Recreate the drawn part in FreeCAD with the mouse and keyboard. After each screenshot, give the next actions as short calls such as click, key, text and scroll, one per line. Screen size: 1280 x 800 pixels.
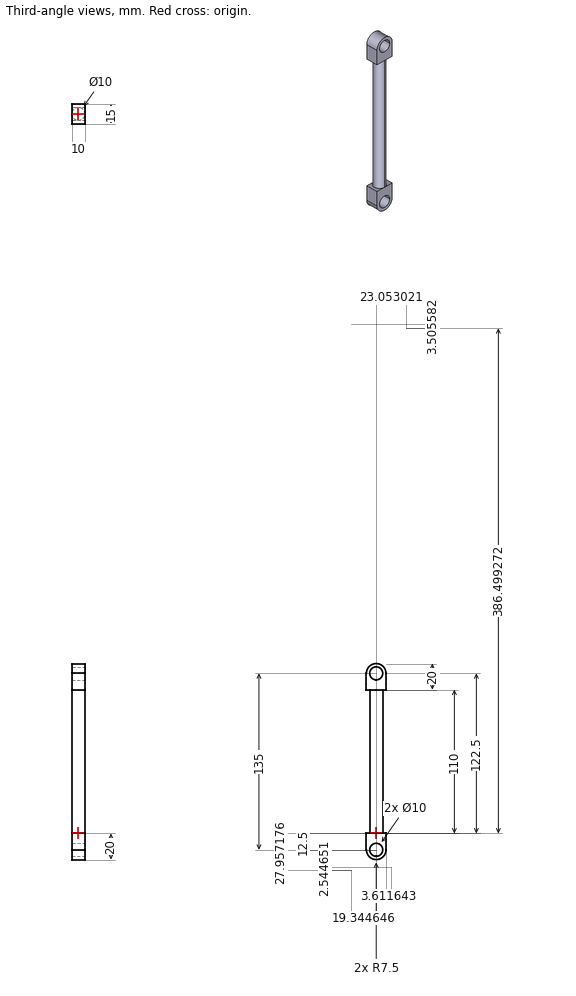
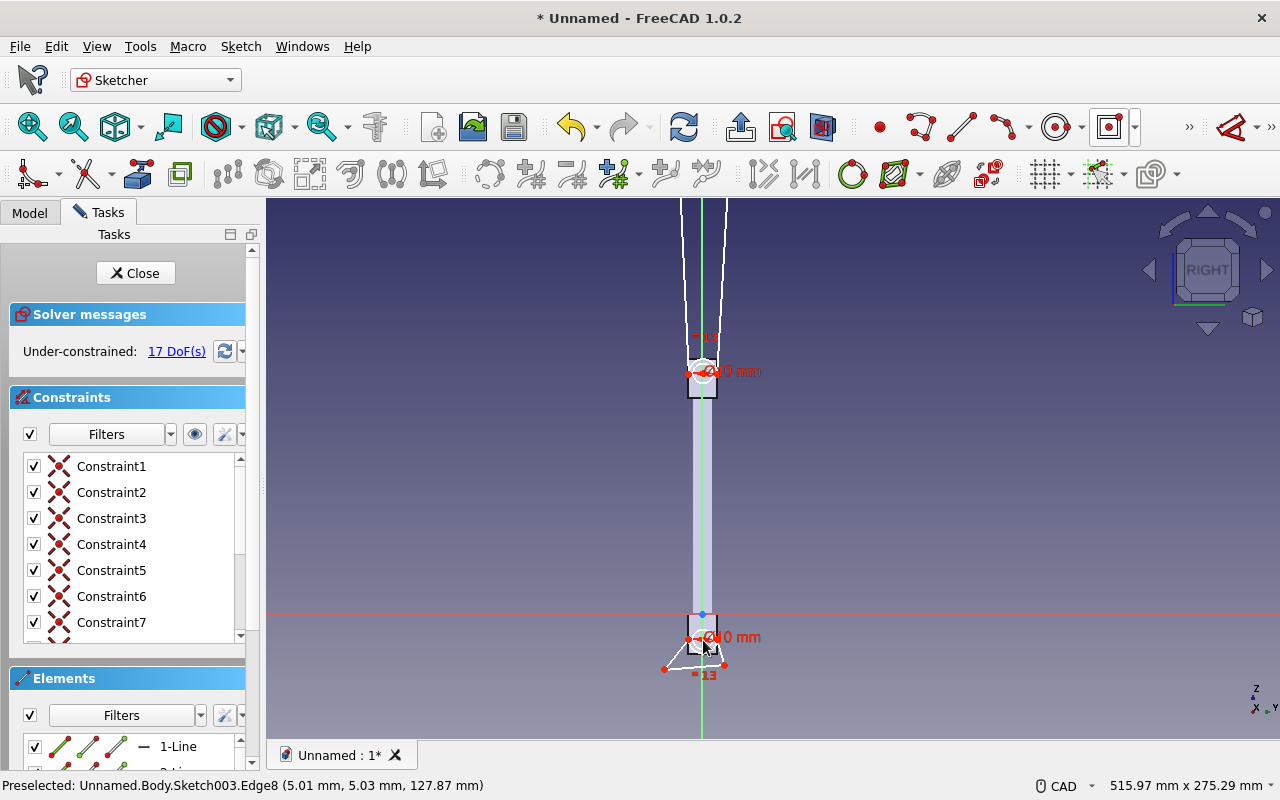
click(703, 639)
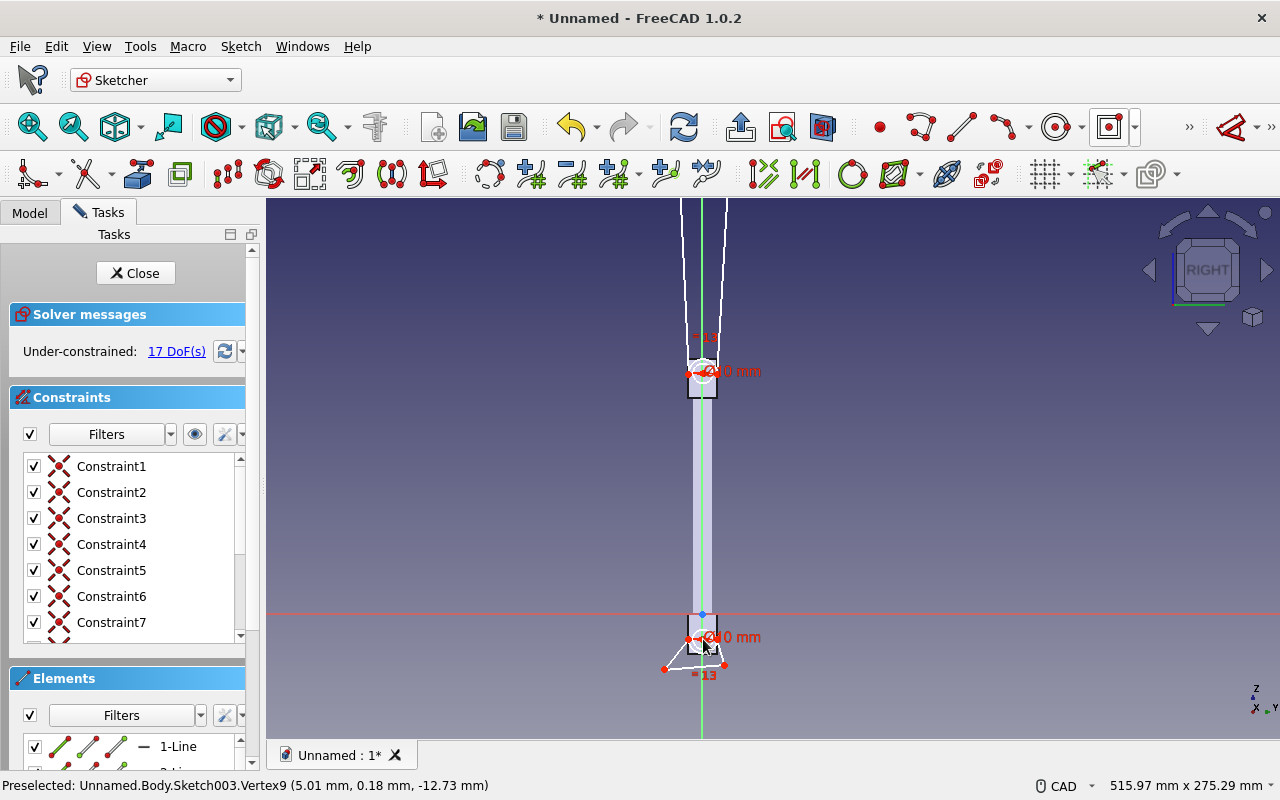
click(702, 572)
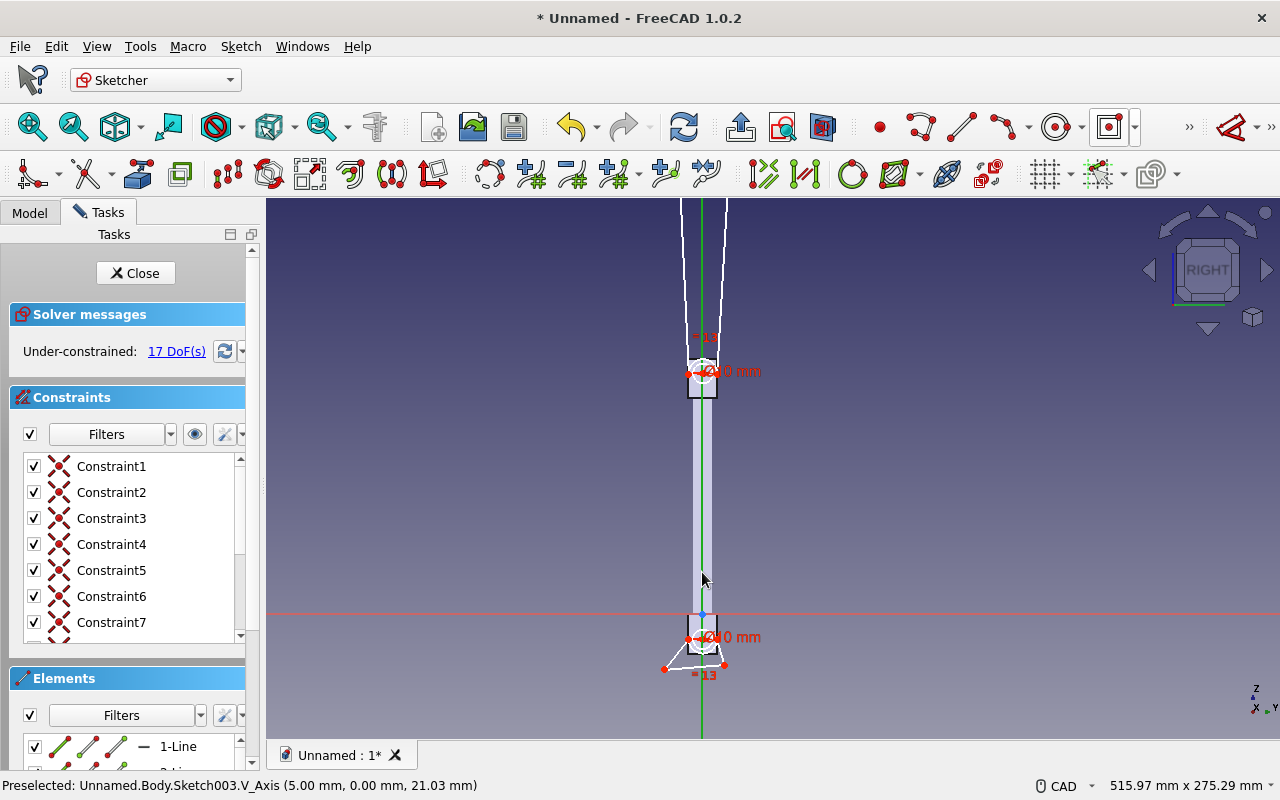
key(c)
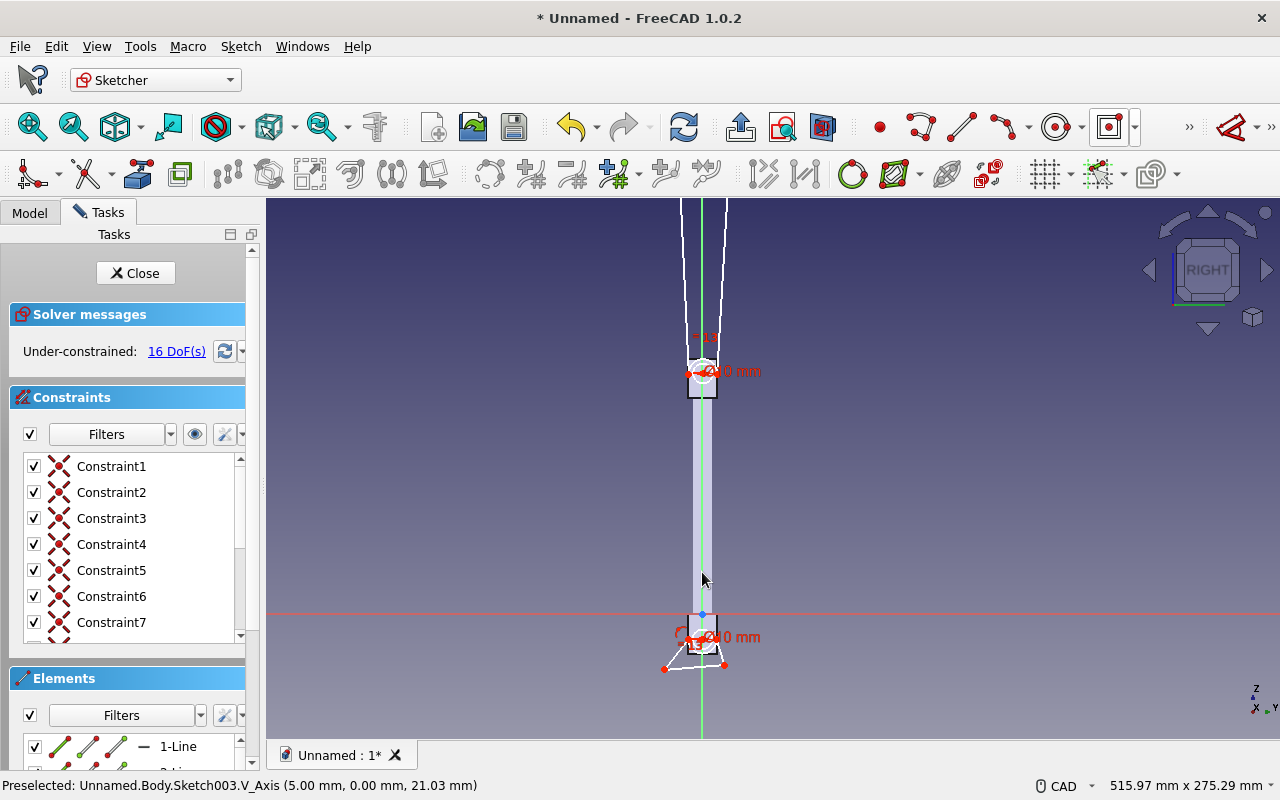
click(703, 373)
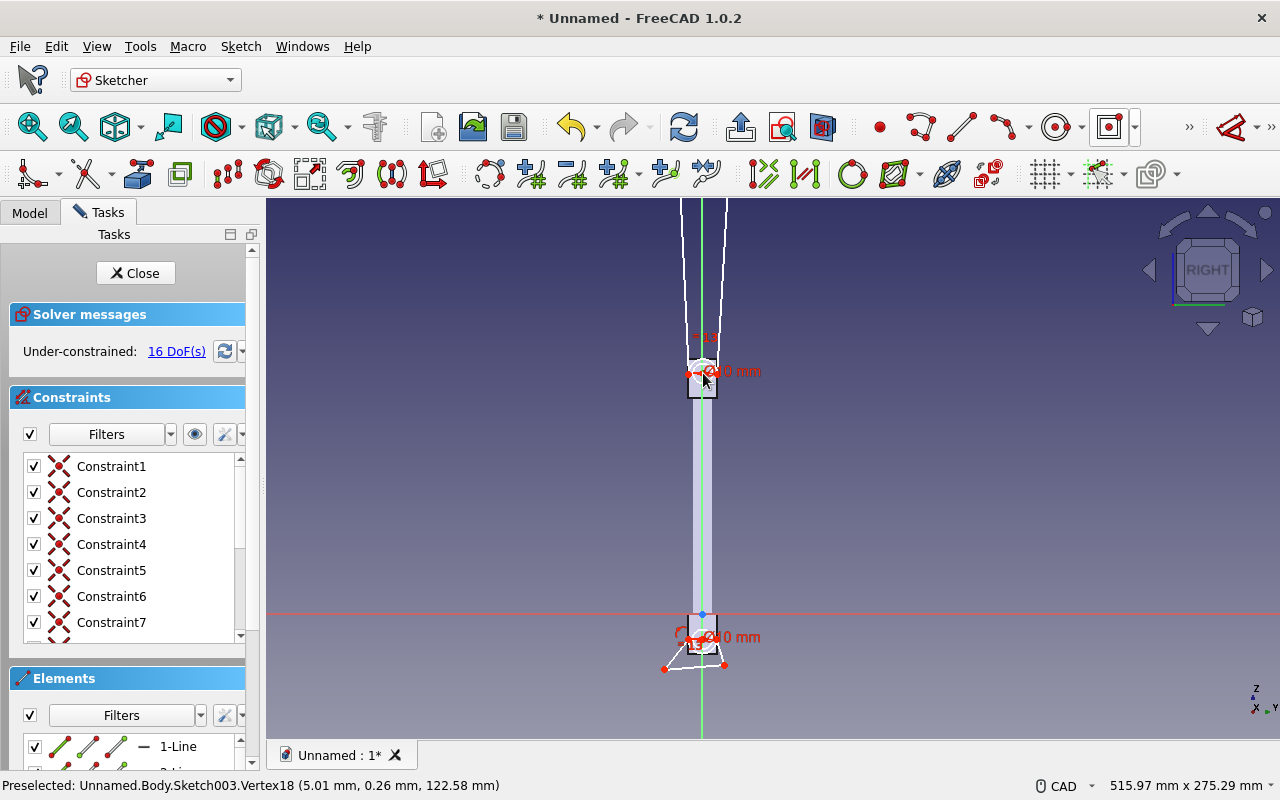
click(702, 572)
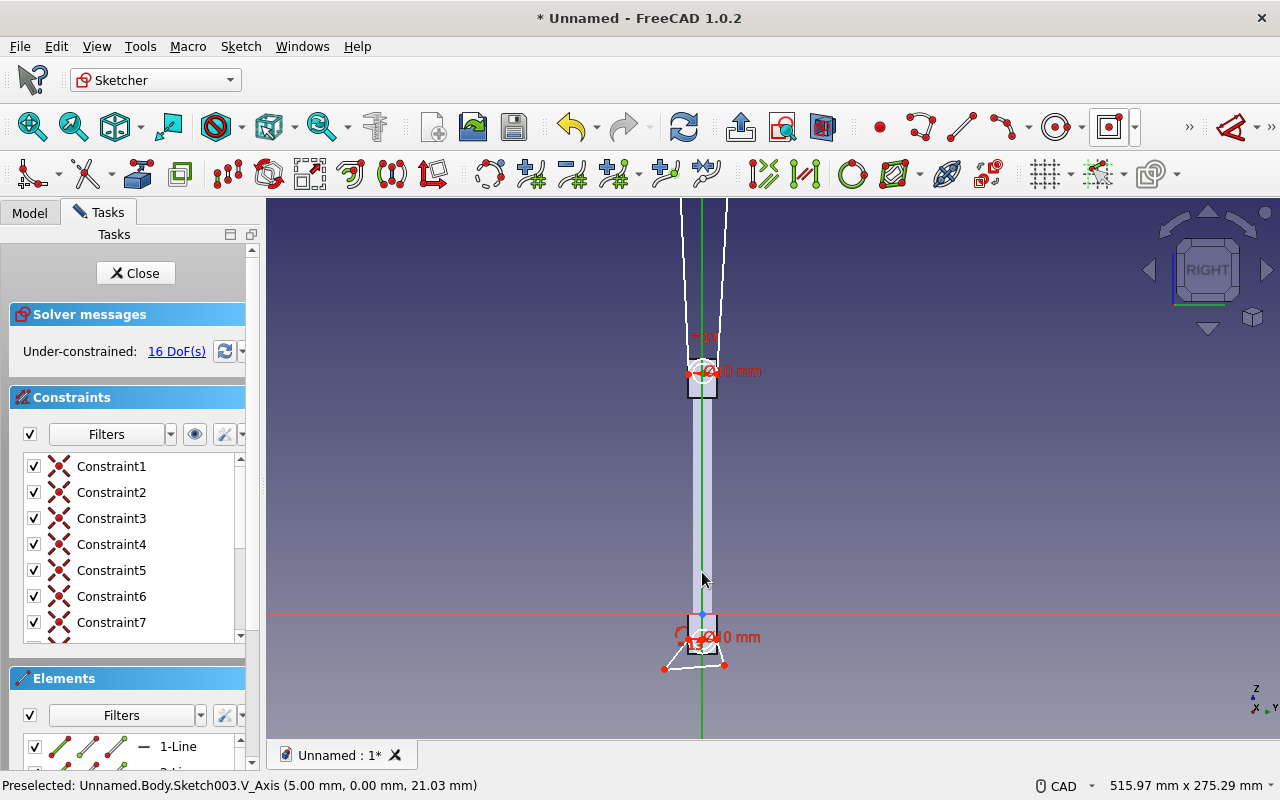
key(c)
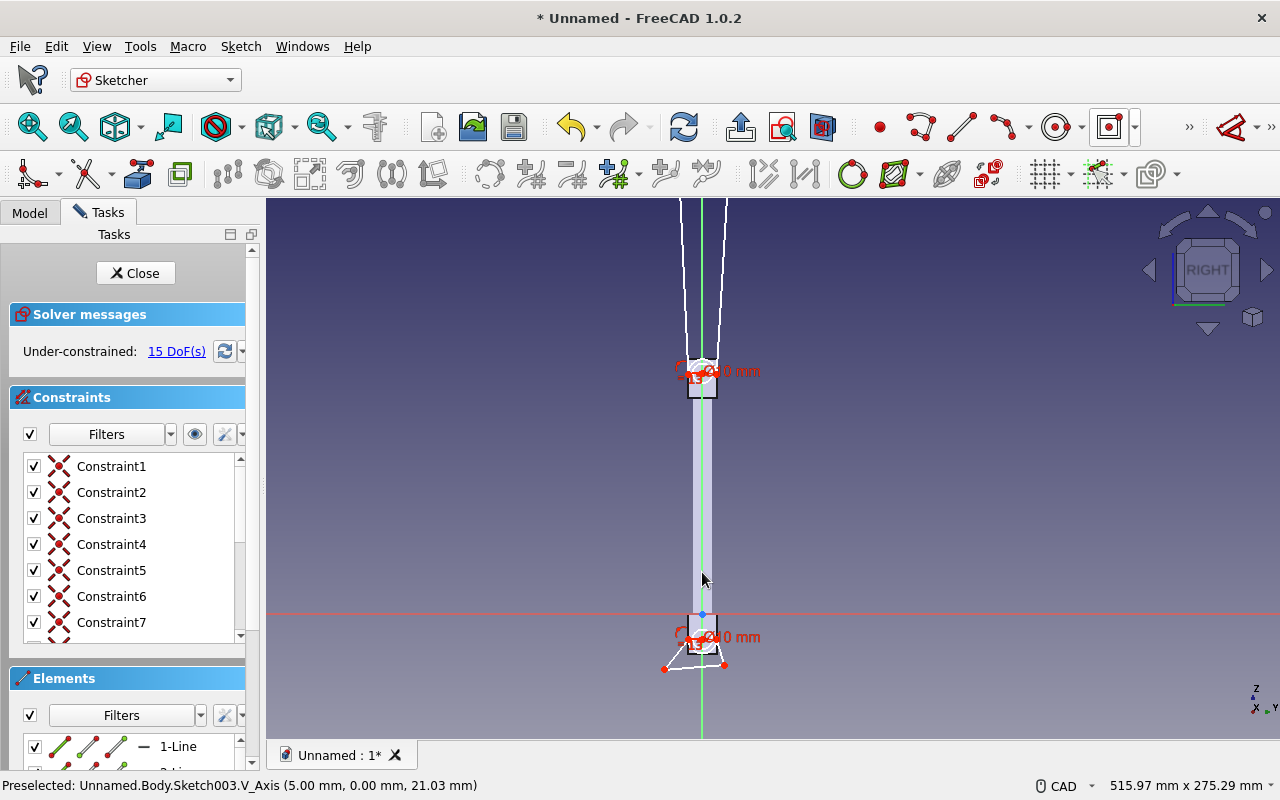
click(1230, 128)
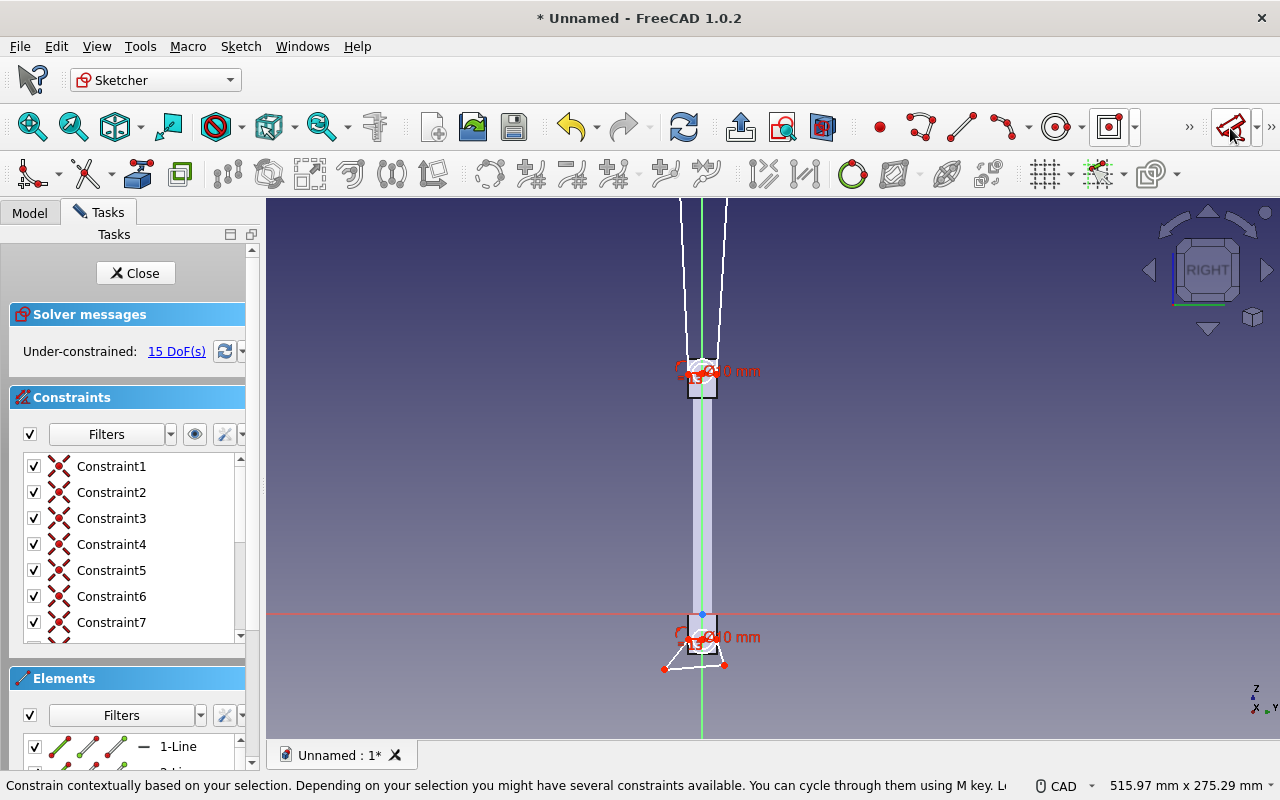
scroll(694, 651, up, 6)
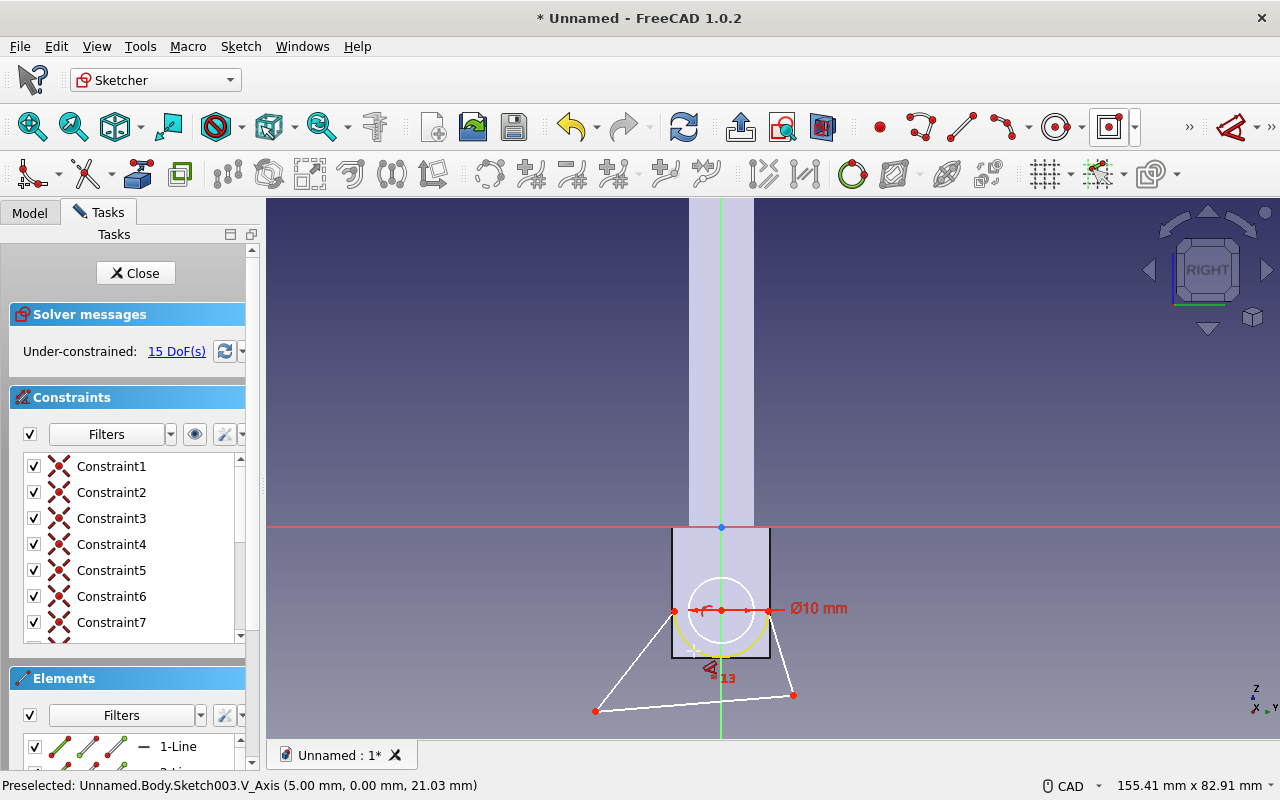
click(694, 649)
click(676, 675)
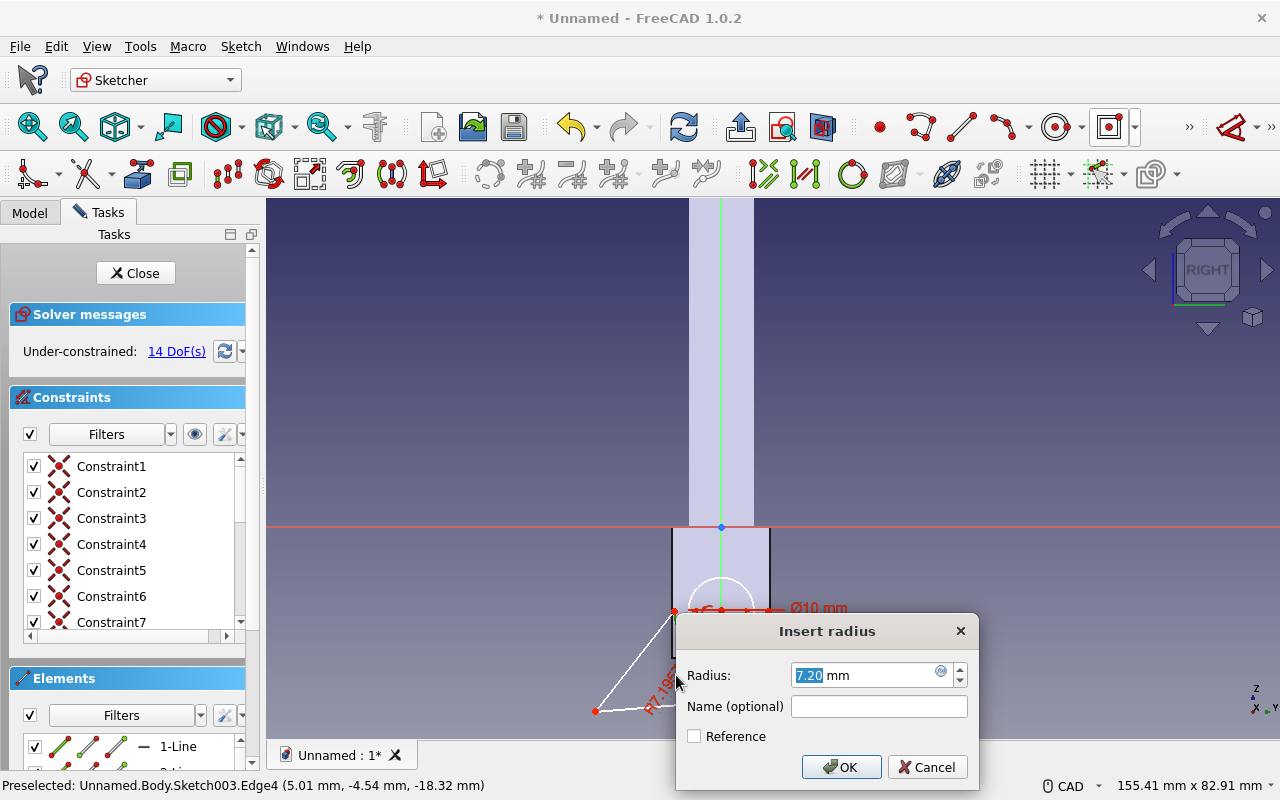
text(7.5)
key(Return)